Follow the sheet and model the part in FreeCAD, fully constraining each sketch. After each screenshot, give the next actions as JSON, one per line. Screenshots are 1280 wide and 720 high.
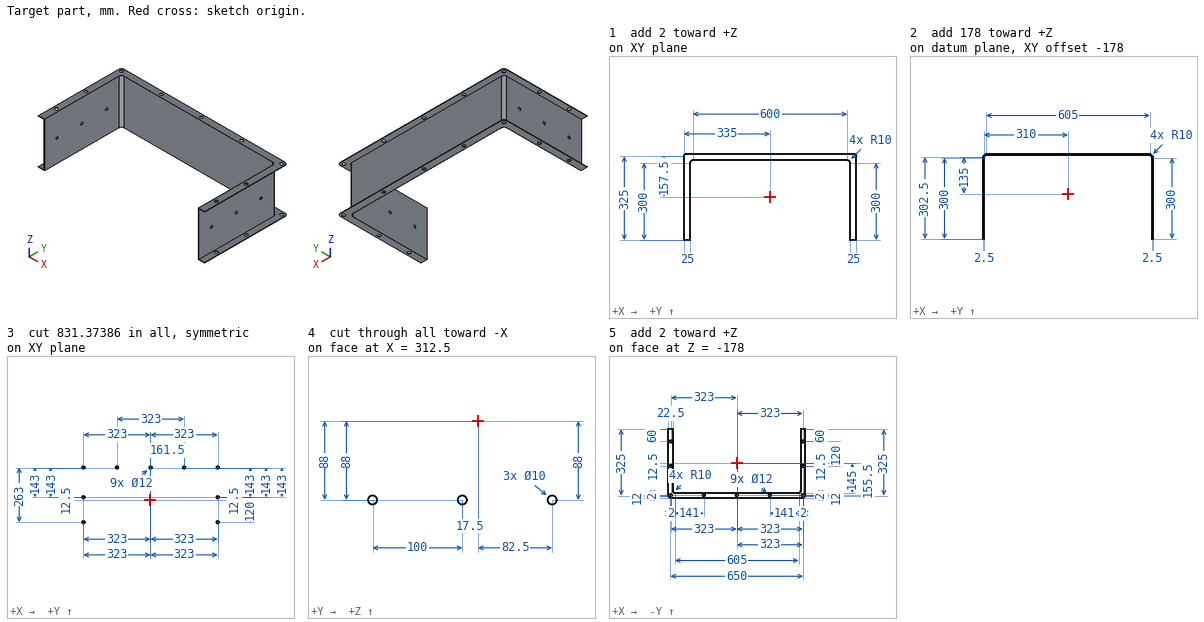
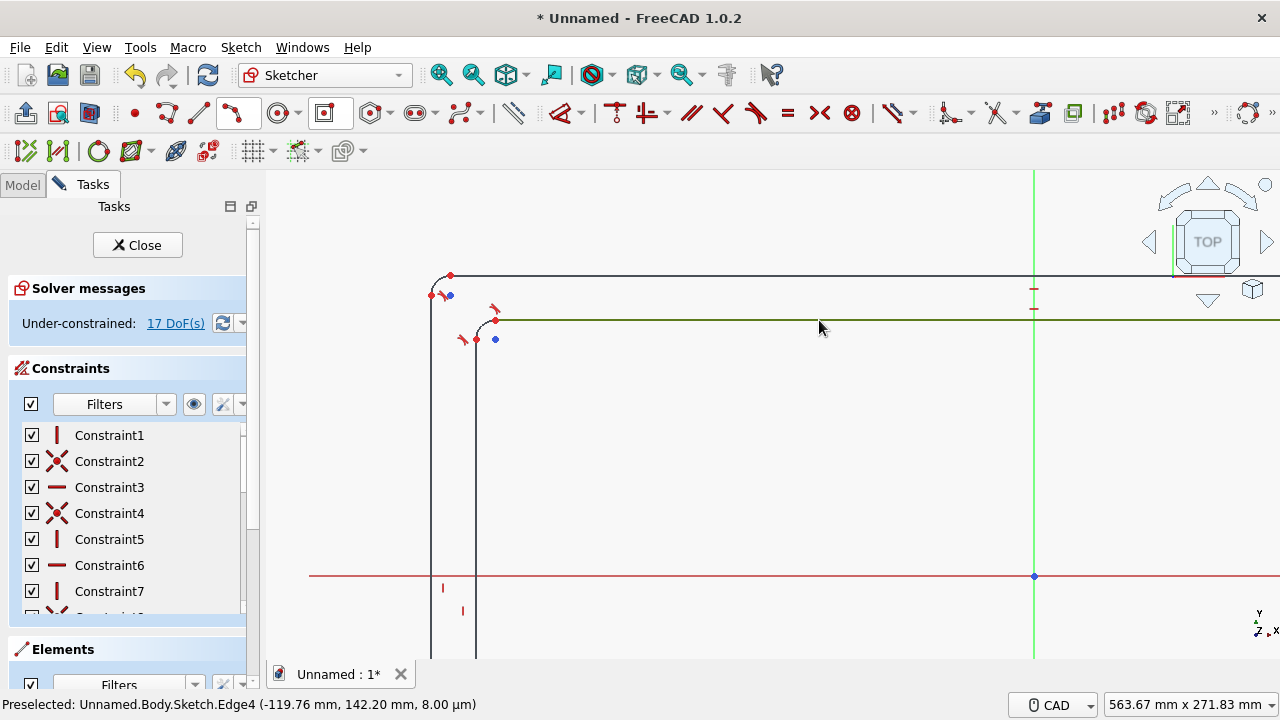
{"action": "scroll", "coordinate": [435, 283], "scroll_direction": "down", "scroll_amount": 4}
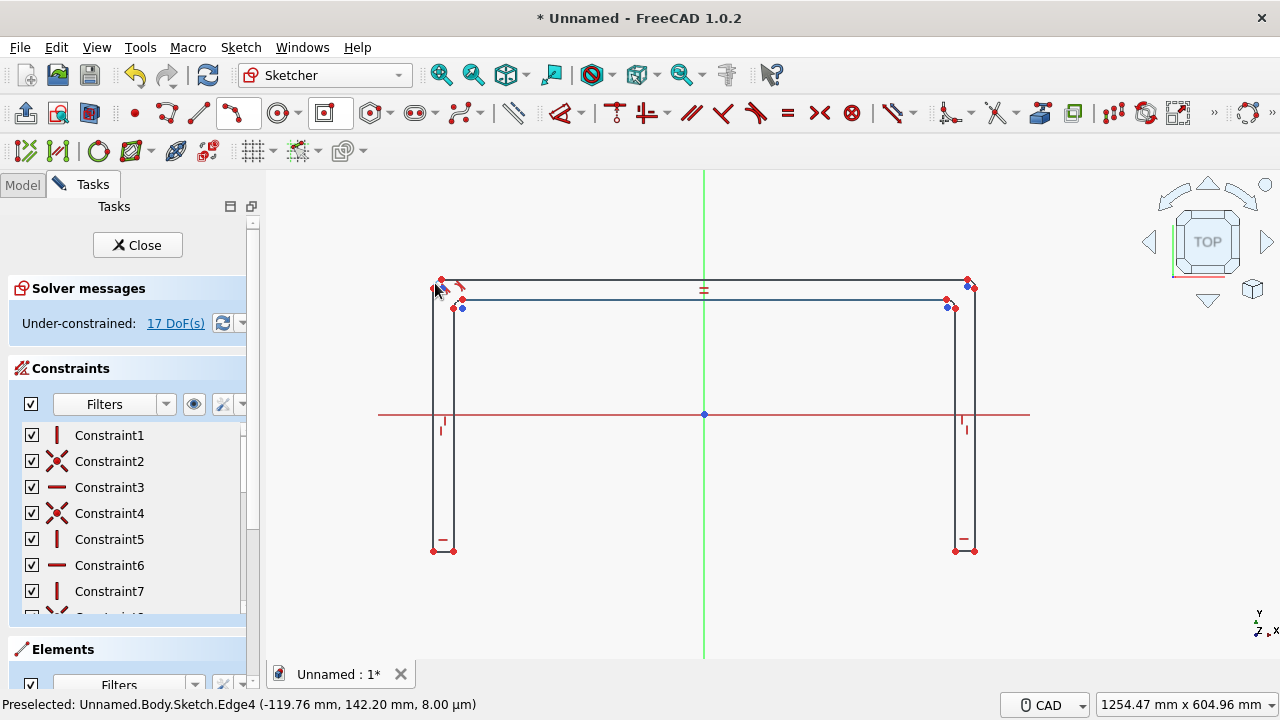
{"action": "scroll", "coordinate": [953, 302], "scroll_direction": "up", "scroll_amount": 4}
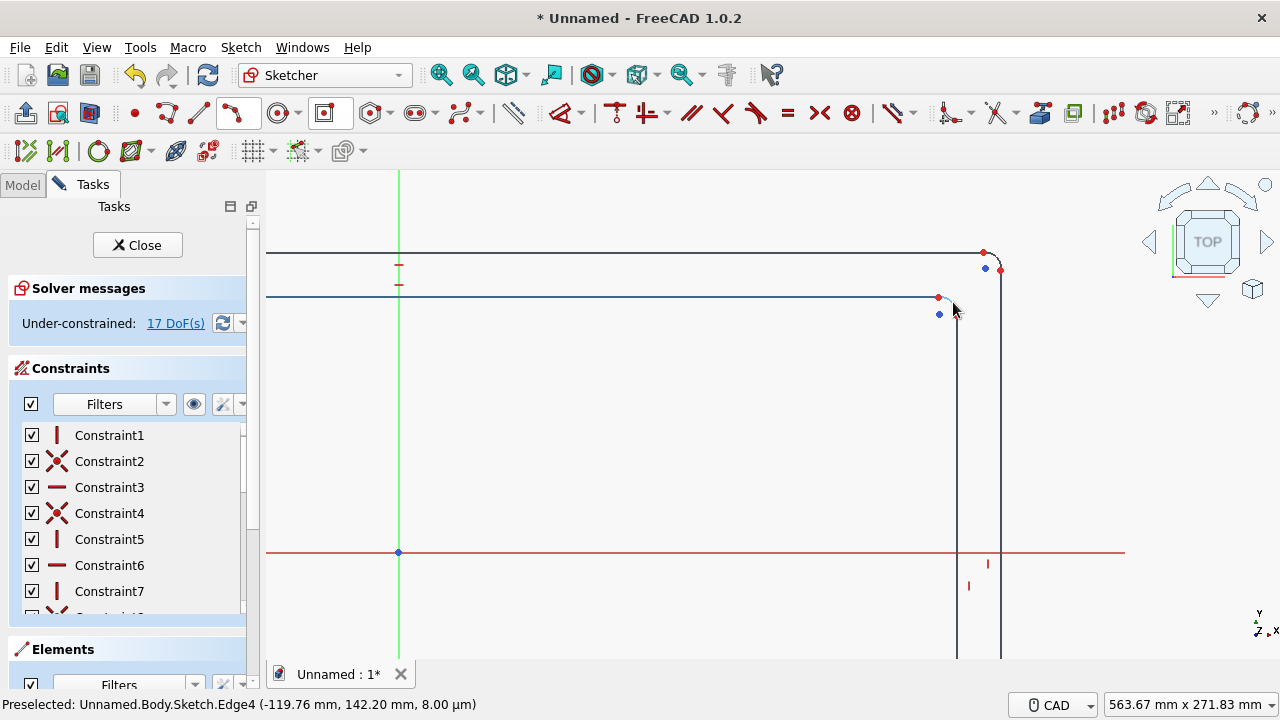
{"action": "left_click", "coordinate": [952, 302]}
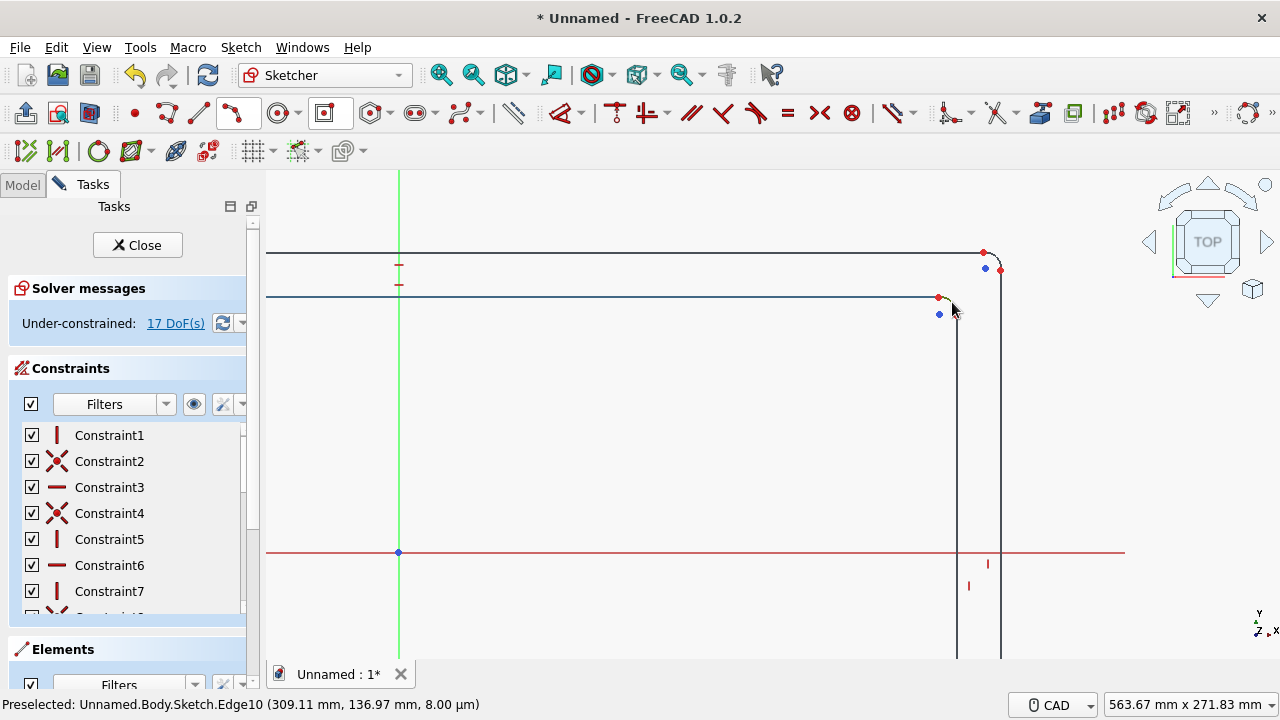
{"action": "left_click", "coordinate": [756, 114]}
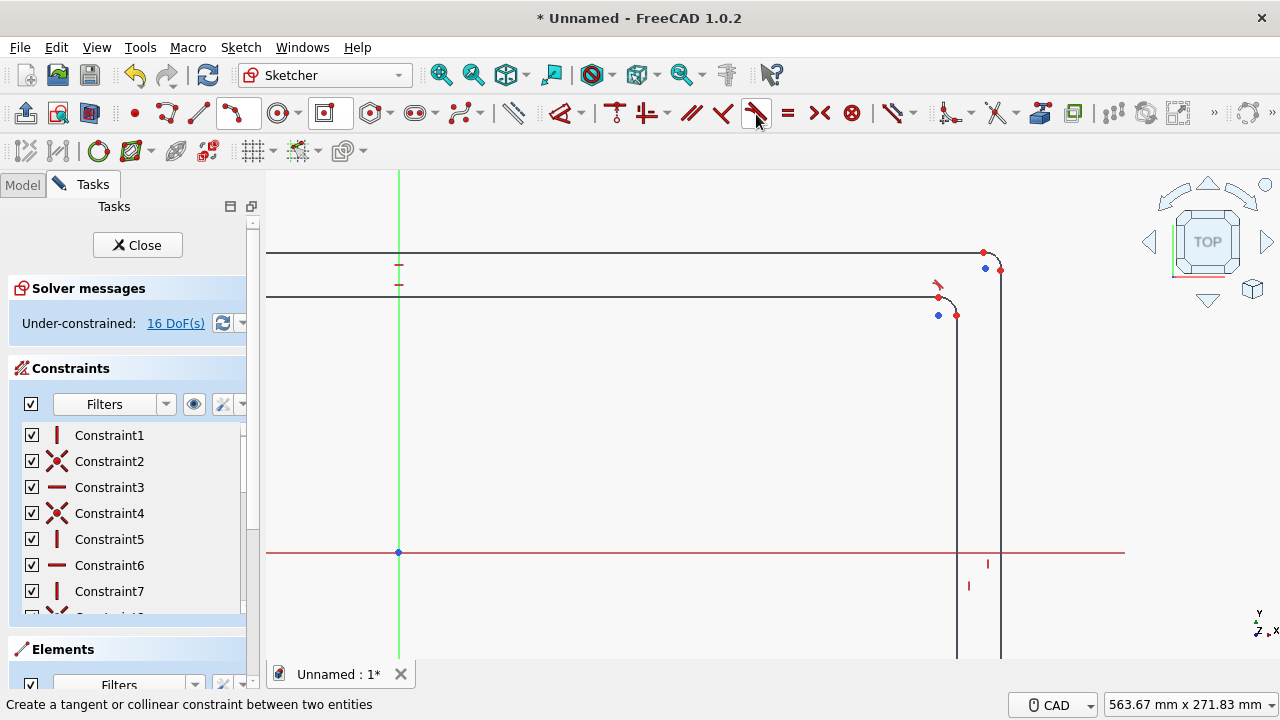
{"action": "left_click", "coordinate": [957, 478]}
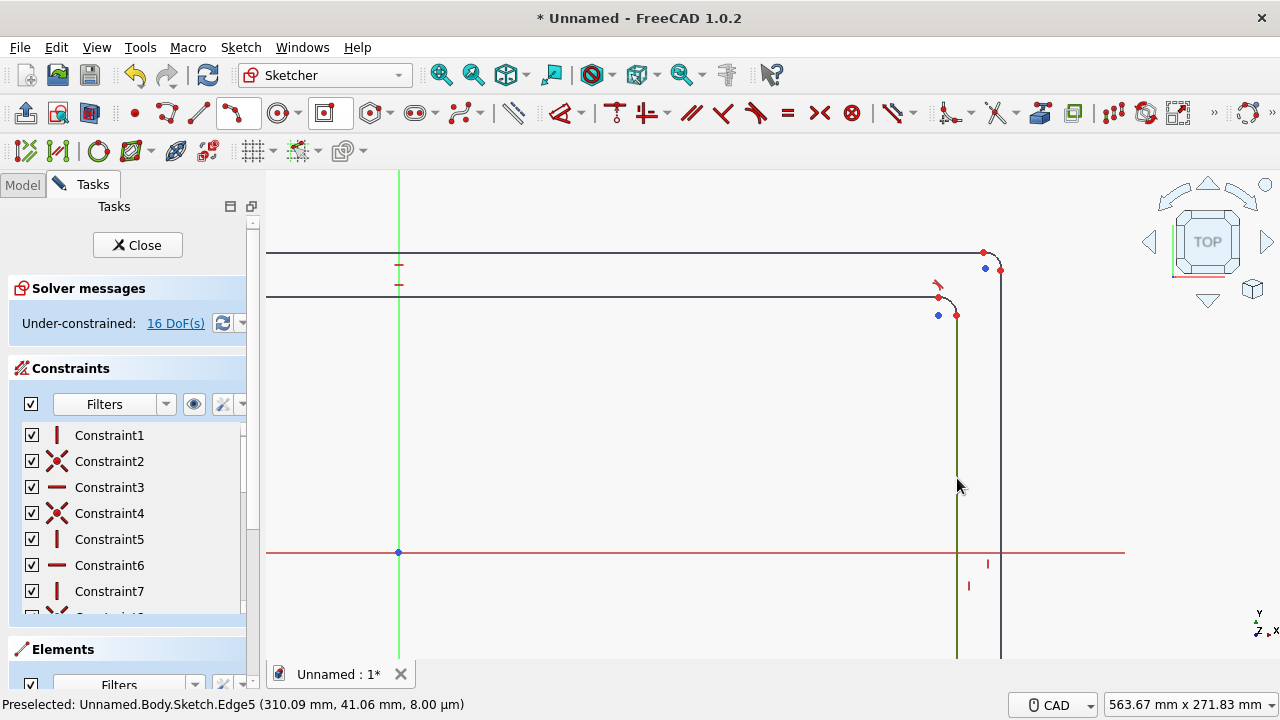
{"action": "left_click", "coordinate": [952, 303]}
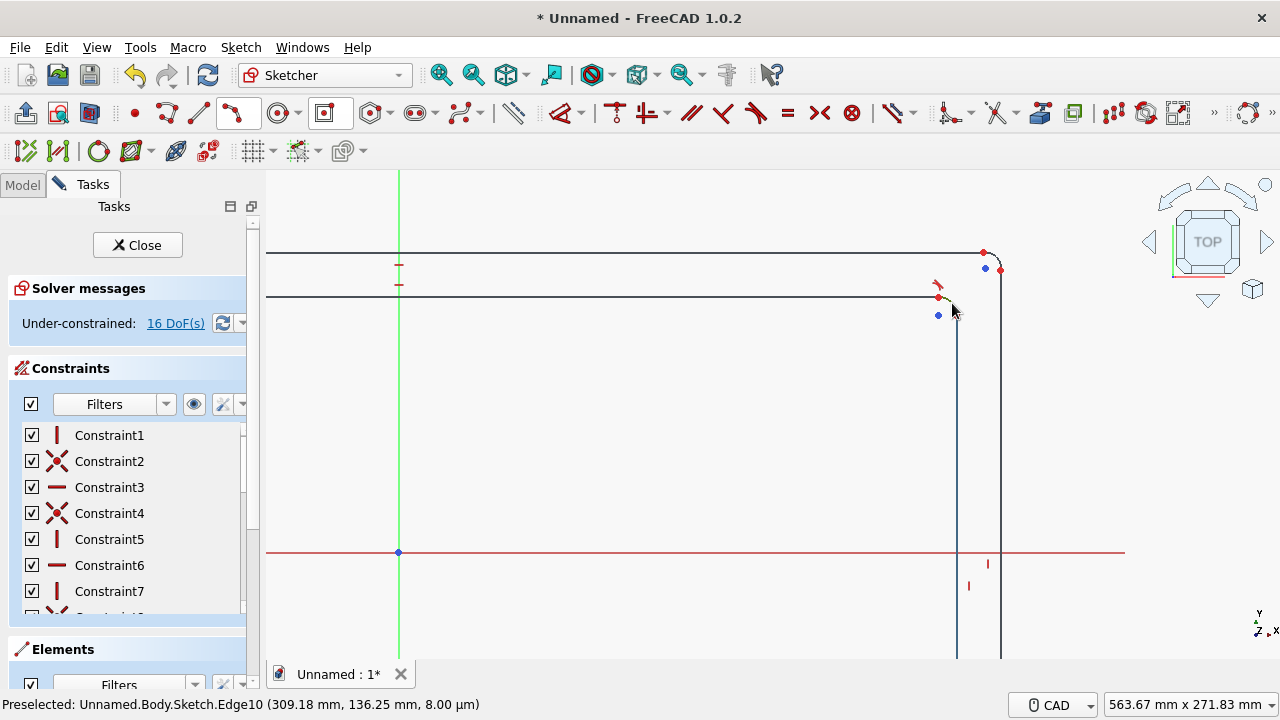
{"action": "key", "text": "t"}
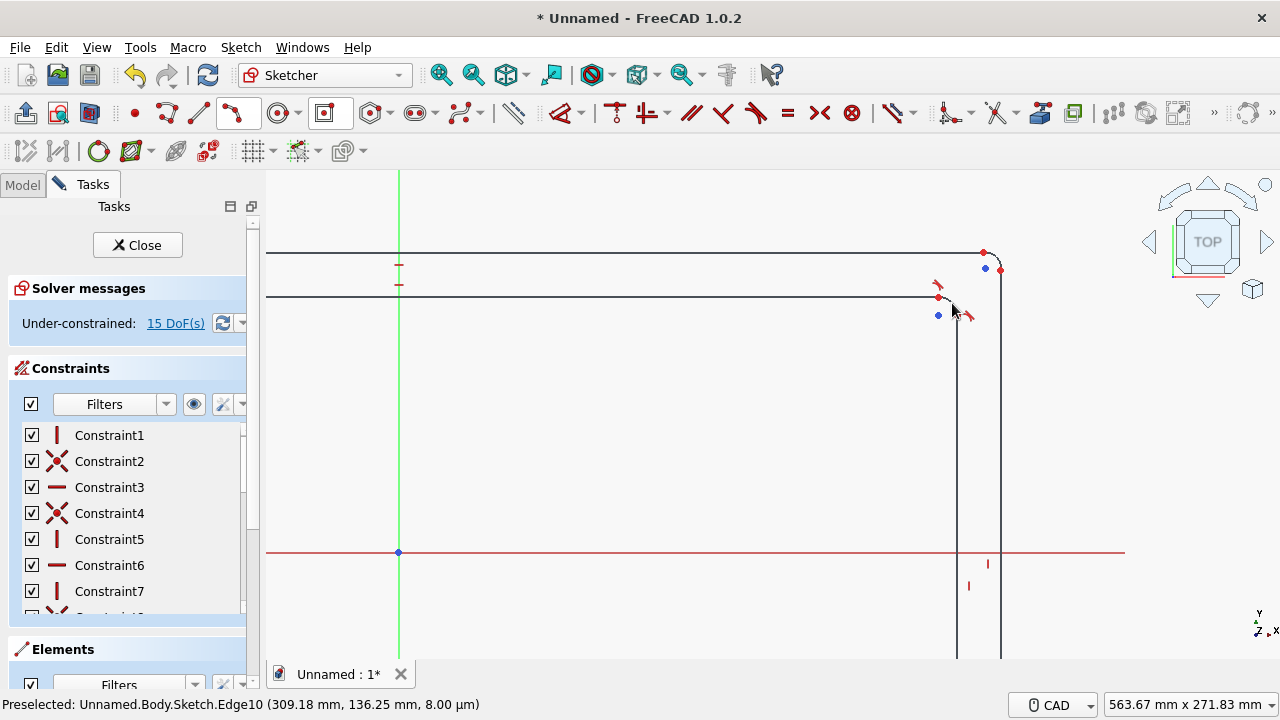
{"action": "left_click", "coordinate": [1001, 447]}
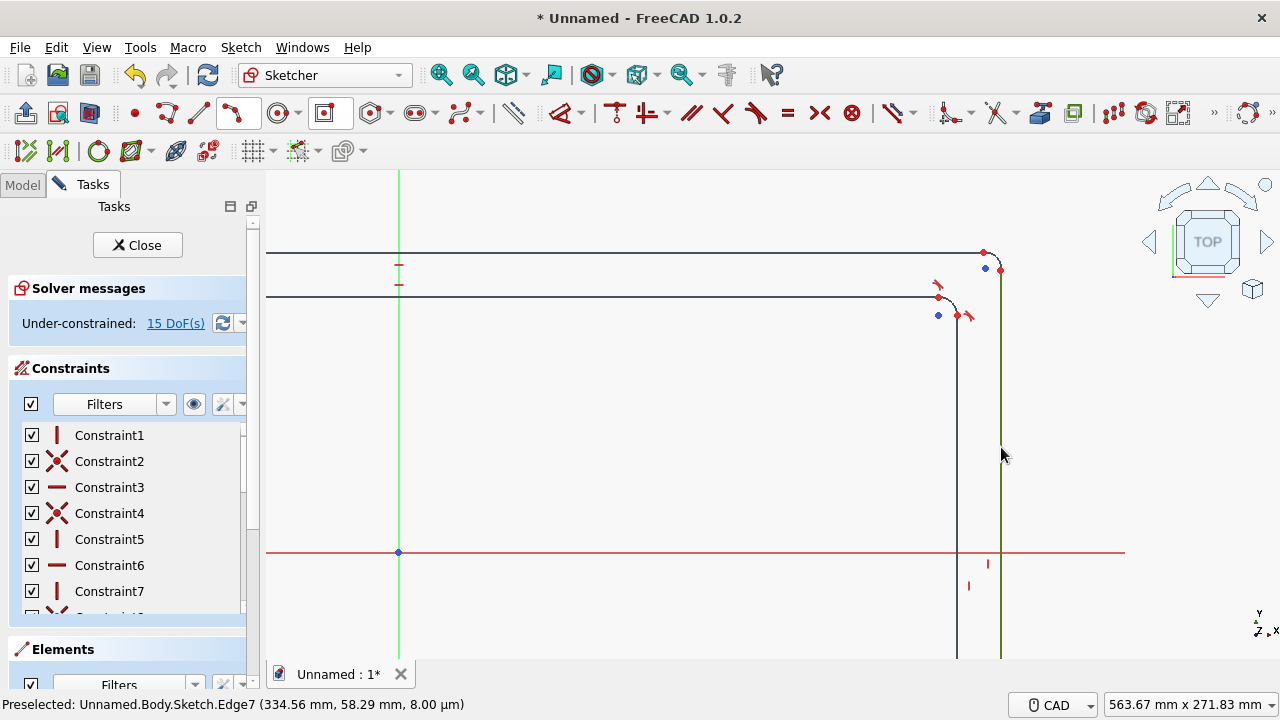
{"action": "left_click", "coordinate": [997, 257]}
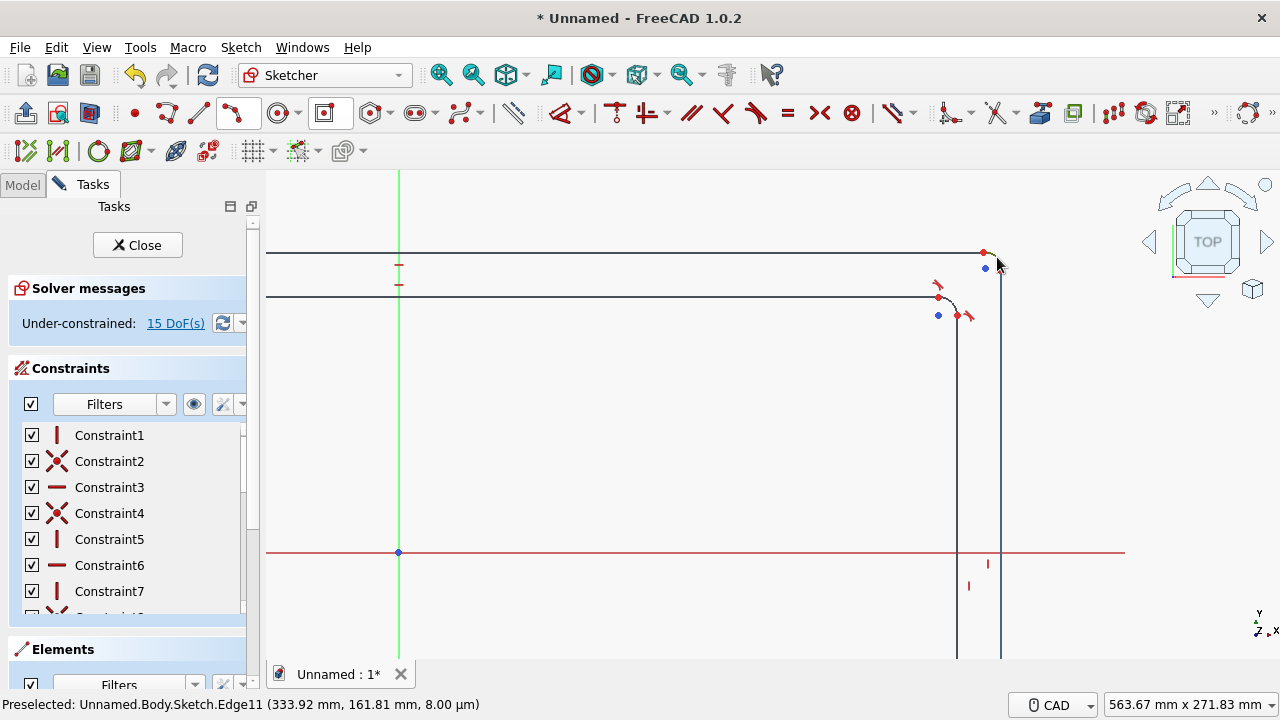
{"action": "left_click", "coordinate": [756, 114]}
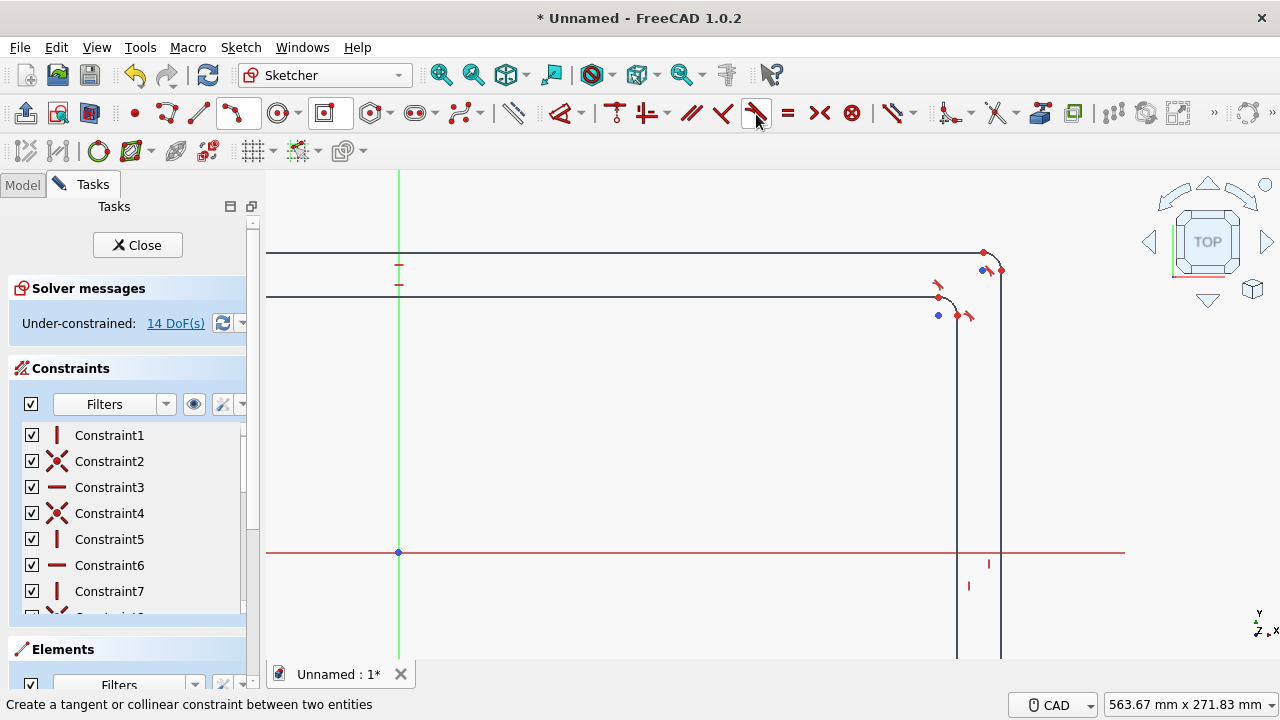
{"action": "left_click", "coordinate": [633, 253]}